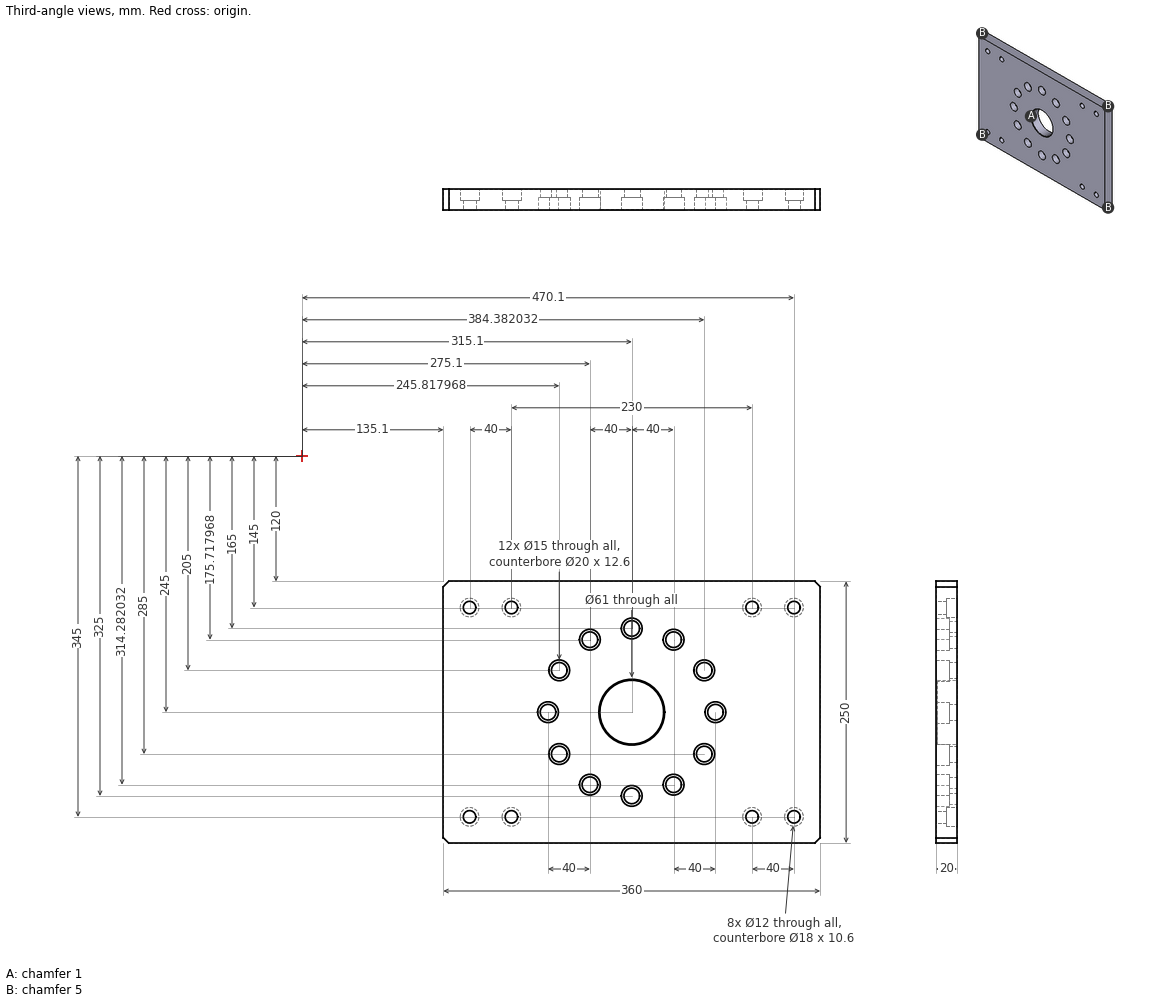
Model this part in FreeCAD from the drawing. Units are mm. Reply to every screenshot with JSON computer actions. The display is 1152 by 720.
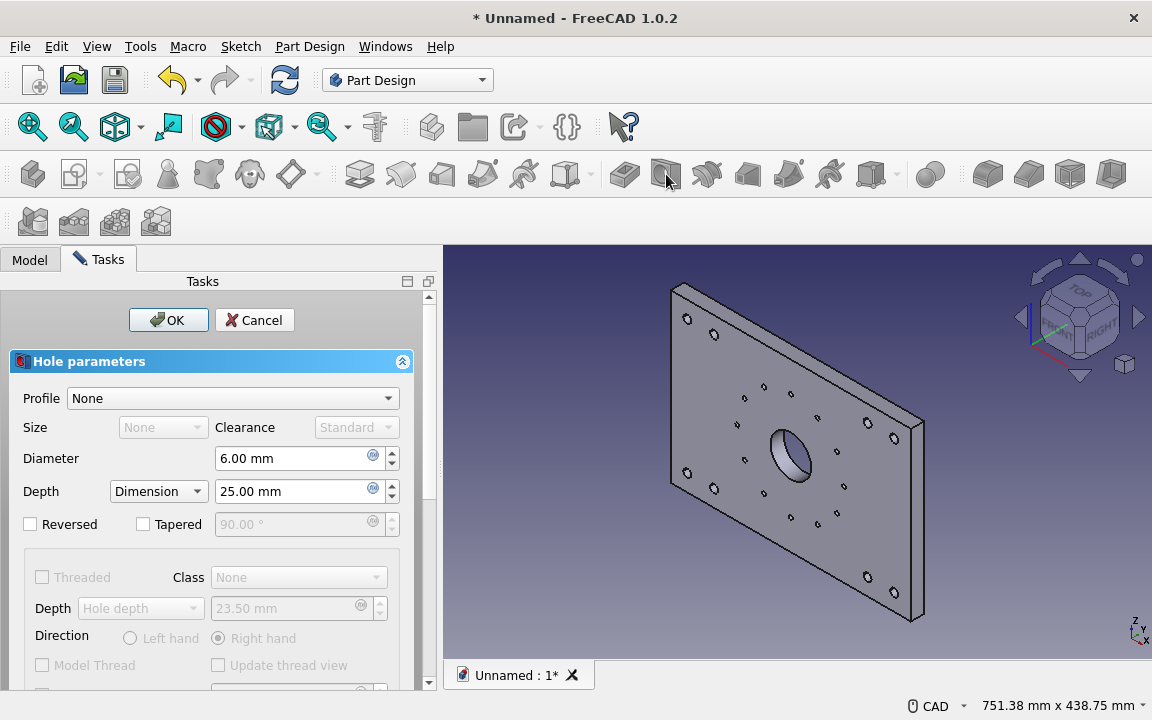
{"action": "triple_click", "coordinate": [300, 458]}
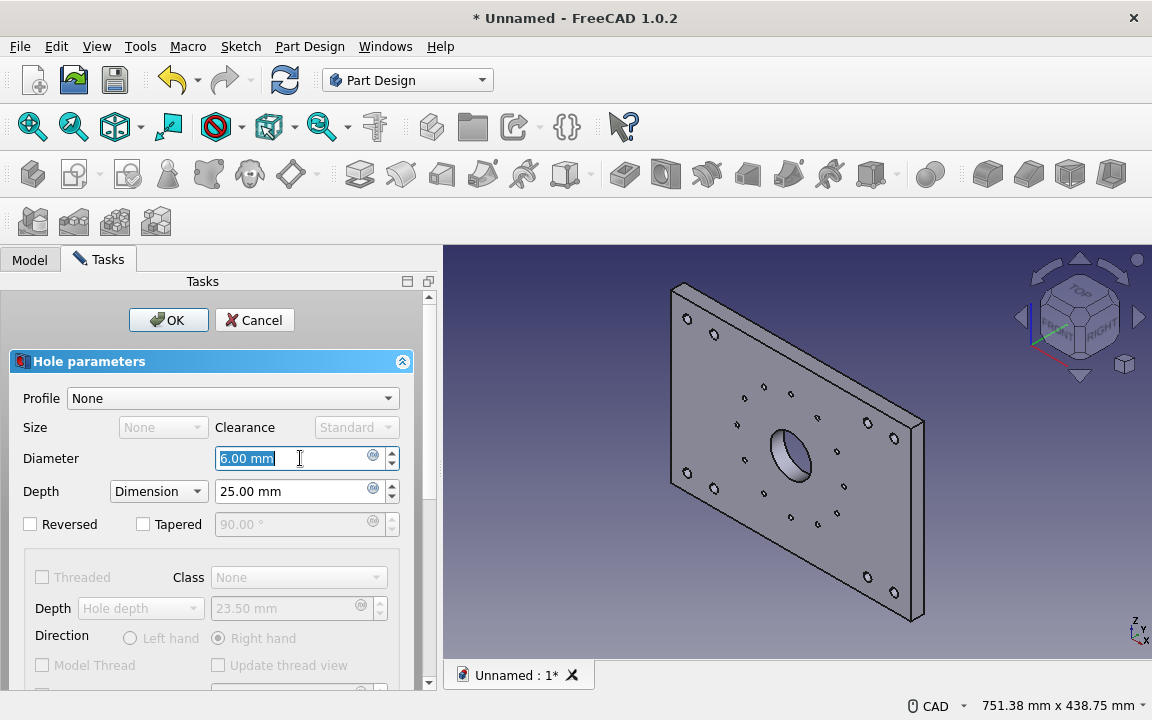
{"action": "type", "text": "15"}
{"action": "key", "text": "Tab"}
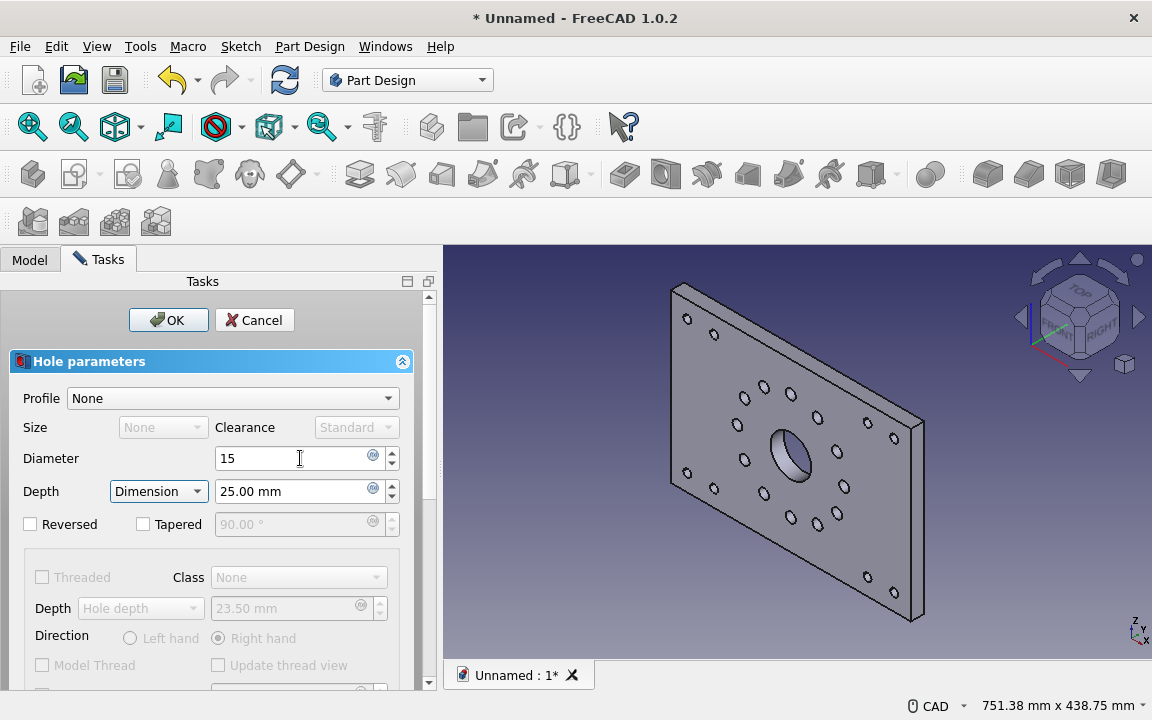
{"action": "left_click", "coordinate": [160, 492]}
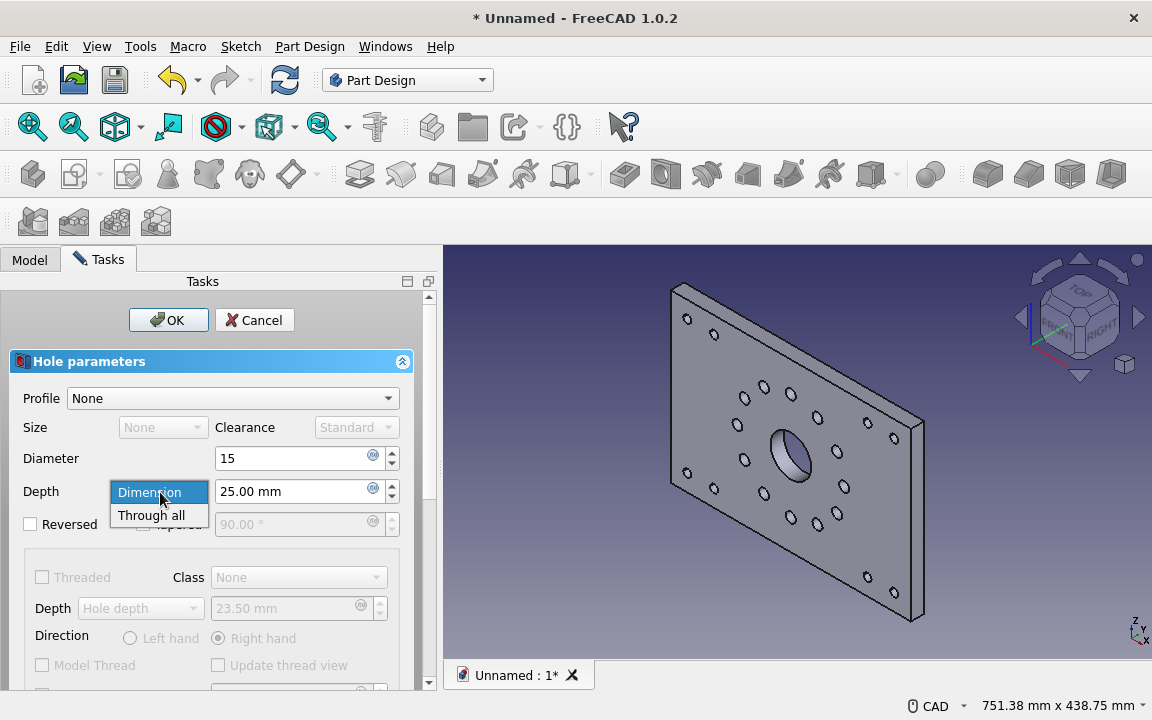
{"action": "left_click", "coordinate": [158, 516]}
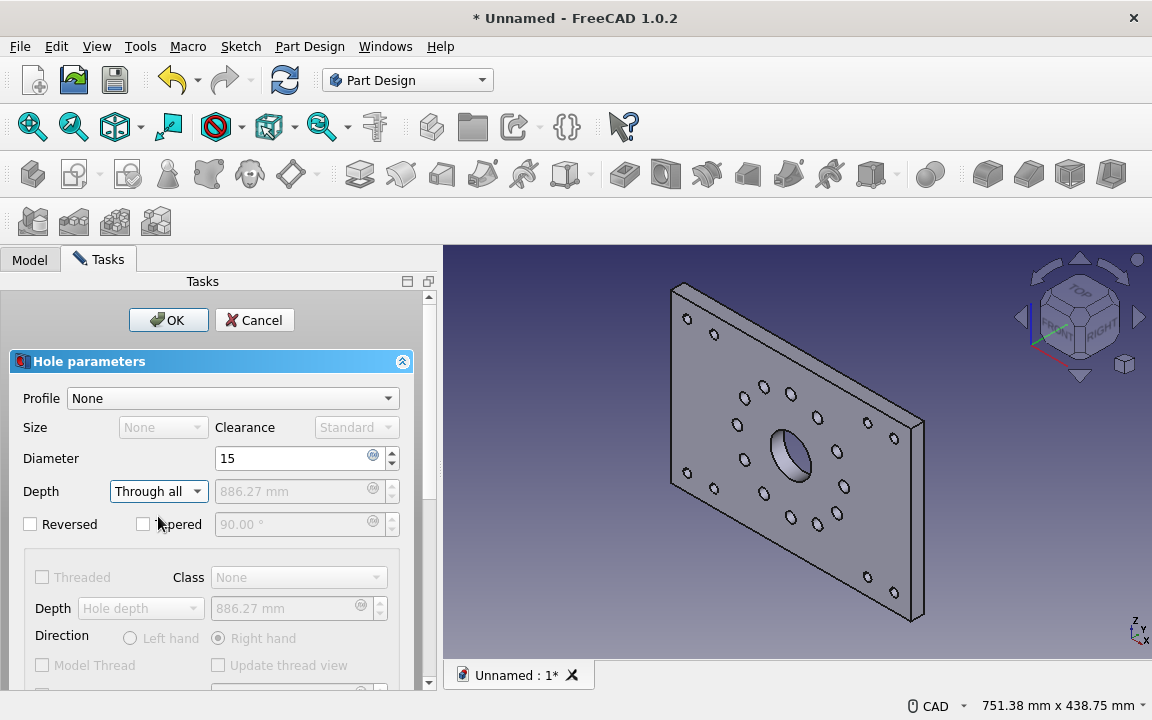
{"action": "scroll", "coordinate": [429, 490], "scroll_direction": "down", "scroll_amount": 3}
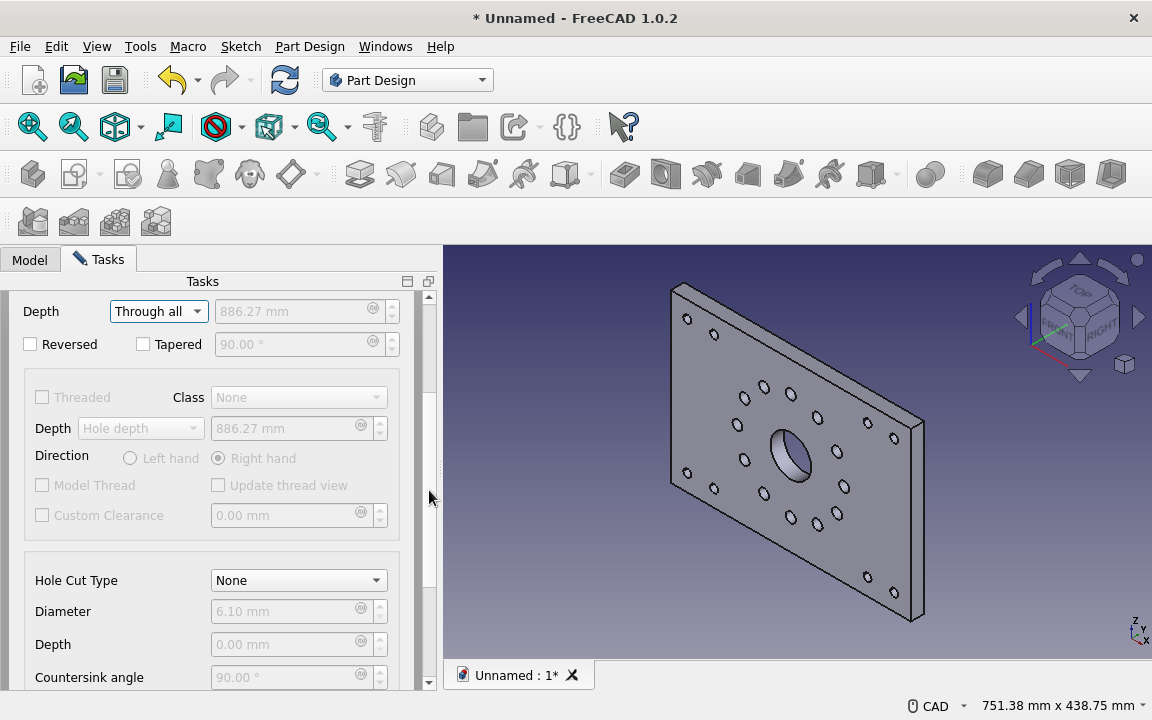
{"action": "left_click", "coordinate": [300, 580]}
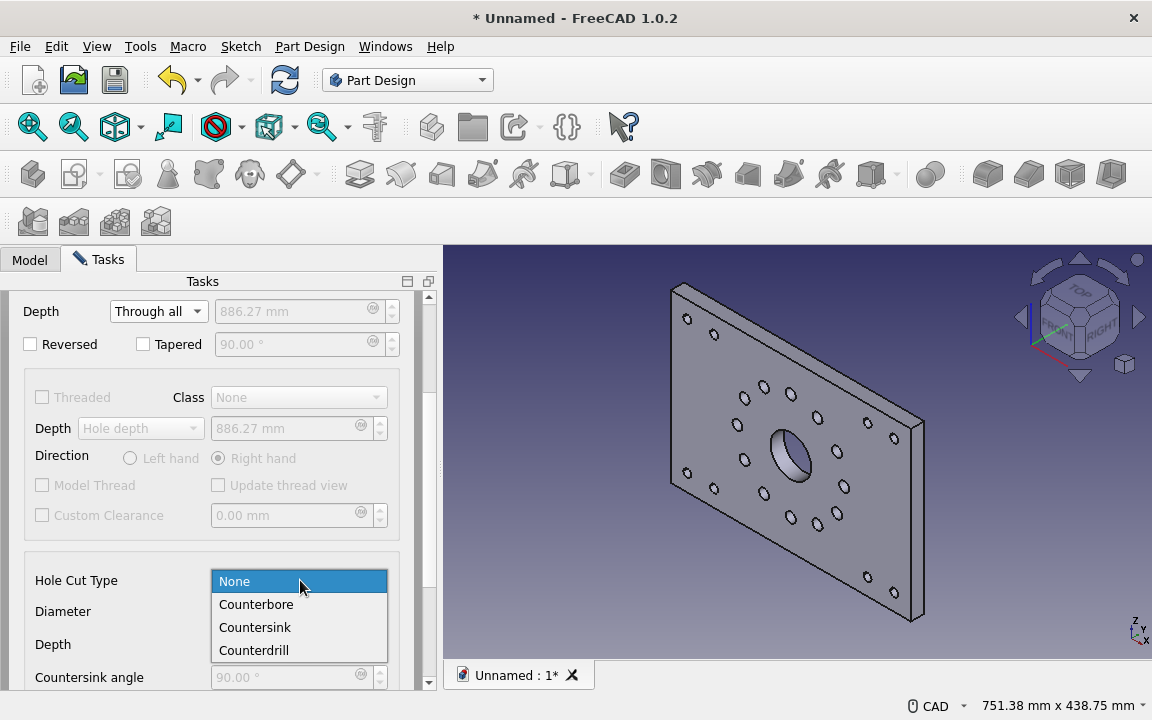
{"action": "left_click", "coordinate": [298, 604]}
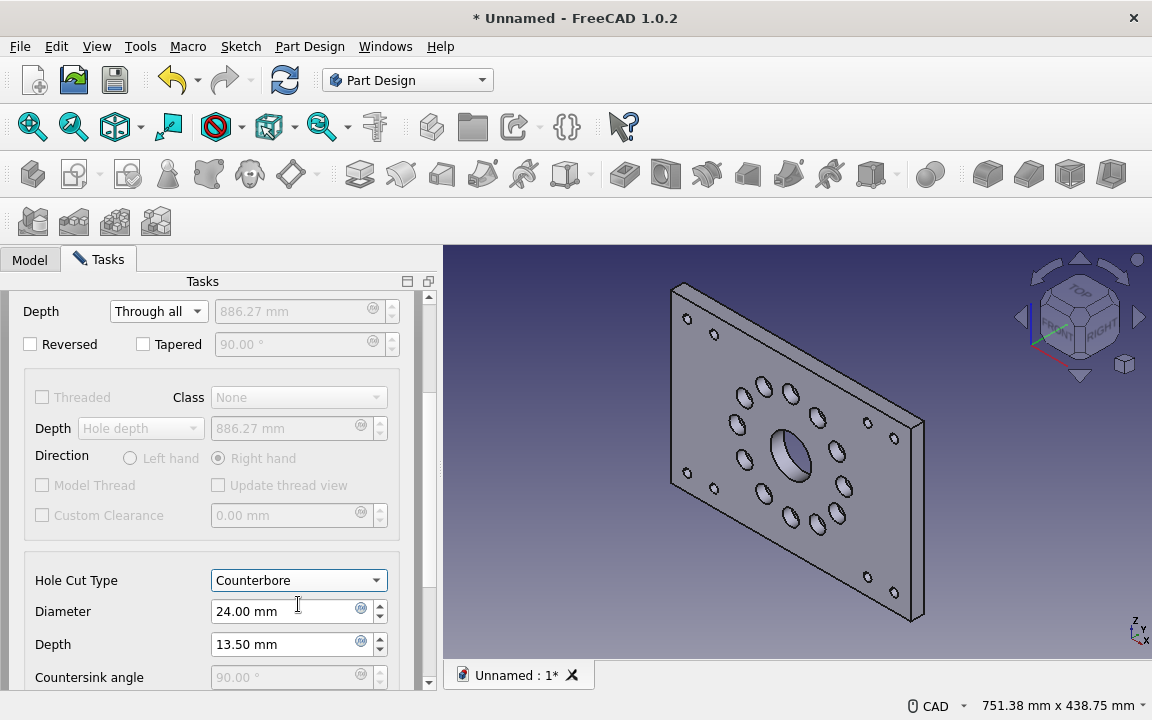
{"action": "triple_click", "coordinate": [292, 612]}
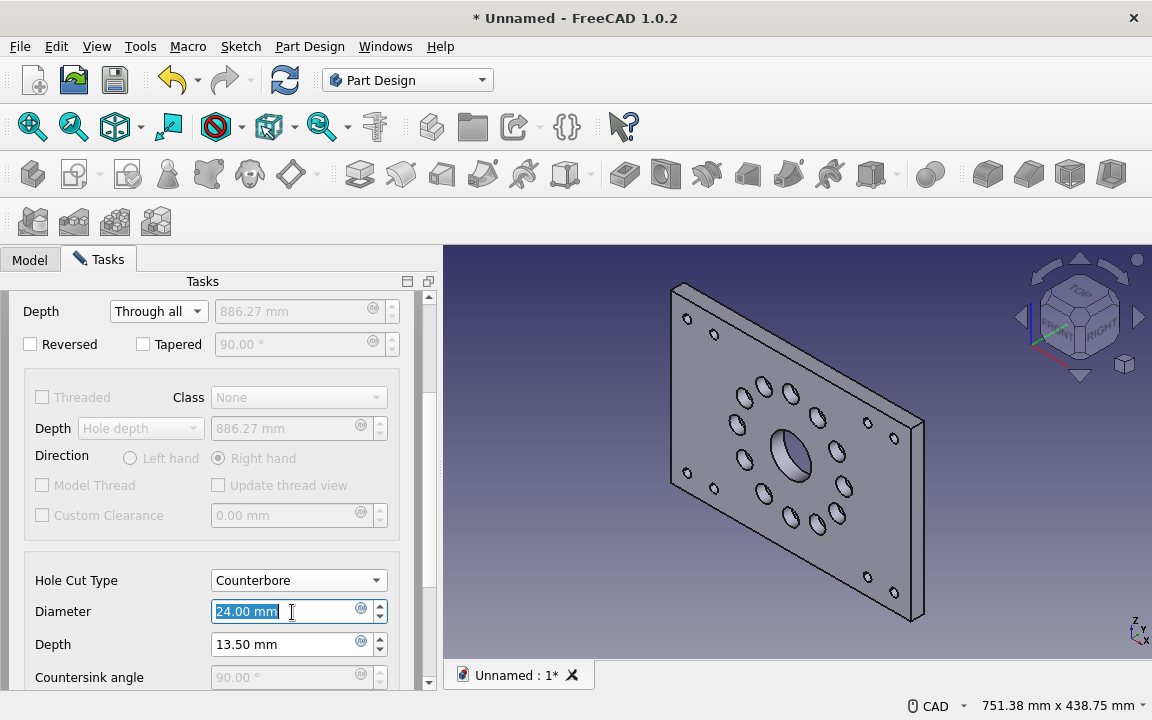
{"action": "type", "text": "20"}
{"action": "key", "text": "Tab"}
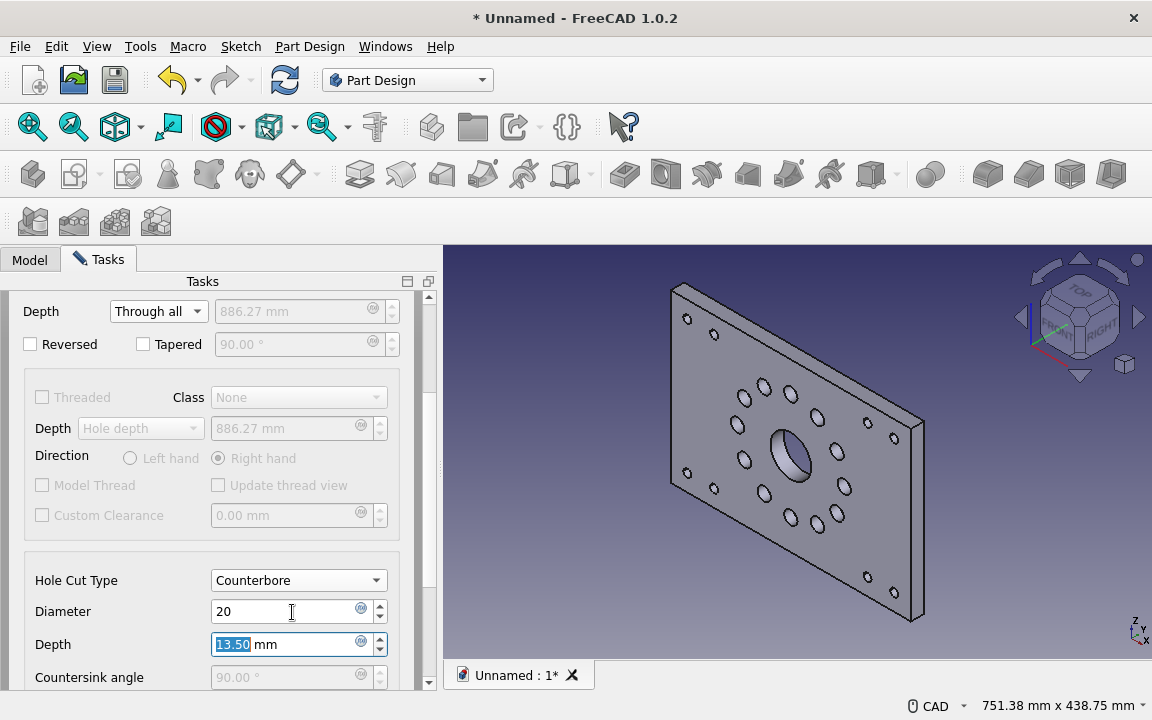
{"action": "type", "text": "12.6"}
{"action": "key", "text": "Tab"}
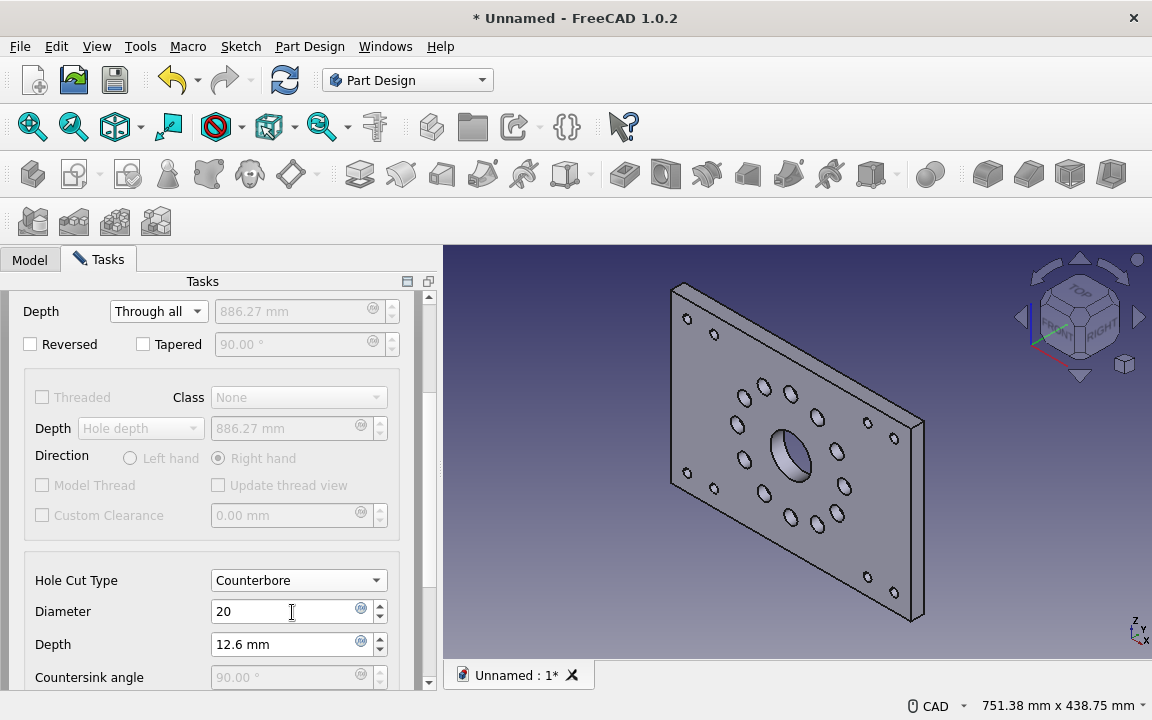
{"action": "scroll", "coordinate": [429, 490], "scroll_direction": "up", "scroll_amount": 4}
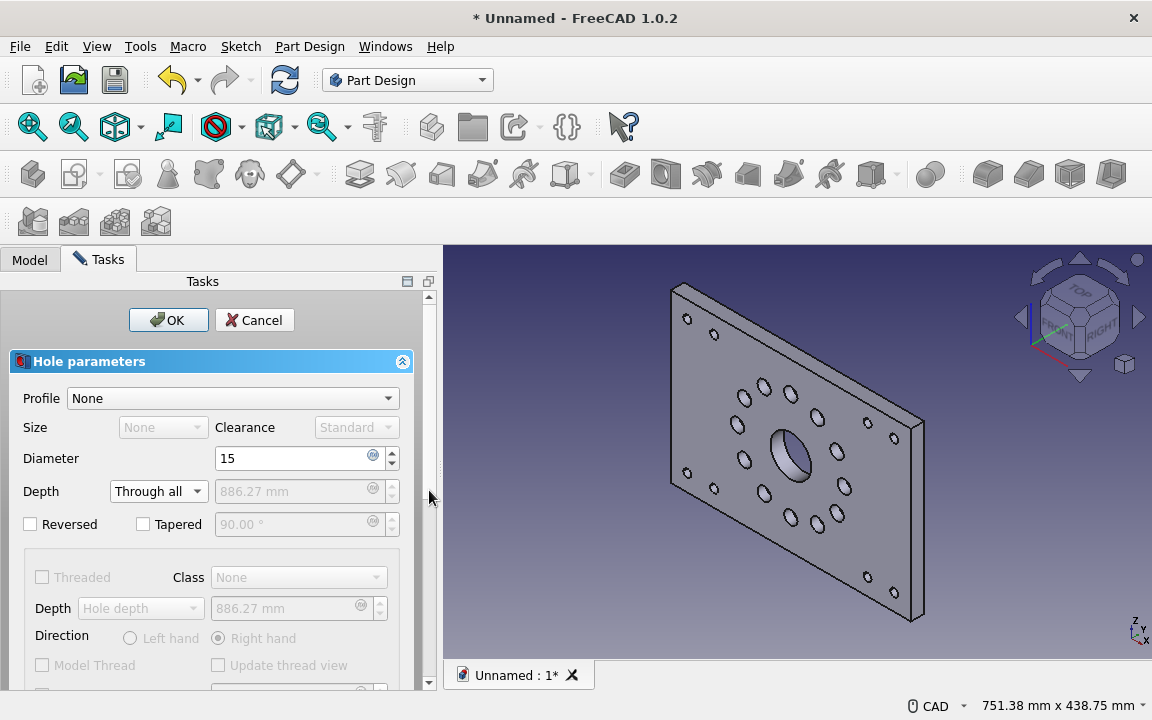
{"action": "left_click", "coordinate": [169, 320]}